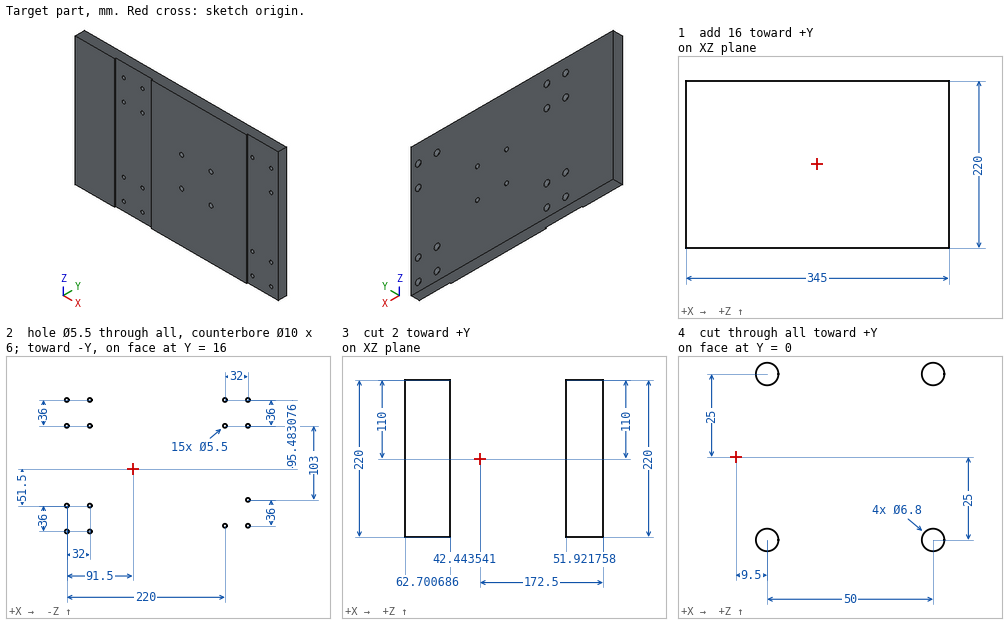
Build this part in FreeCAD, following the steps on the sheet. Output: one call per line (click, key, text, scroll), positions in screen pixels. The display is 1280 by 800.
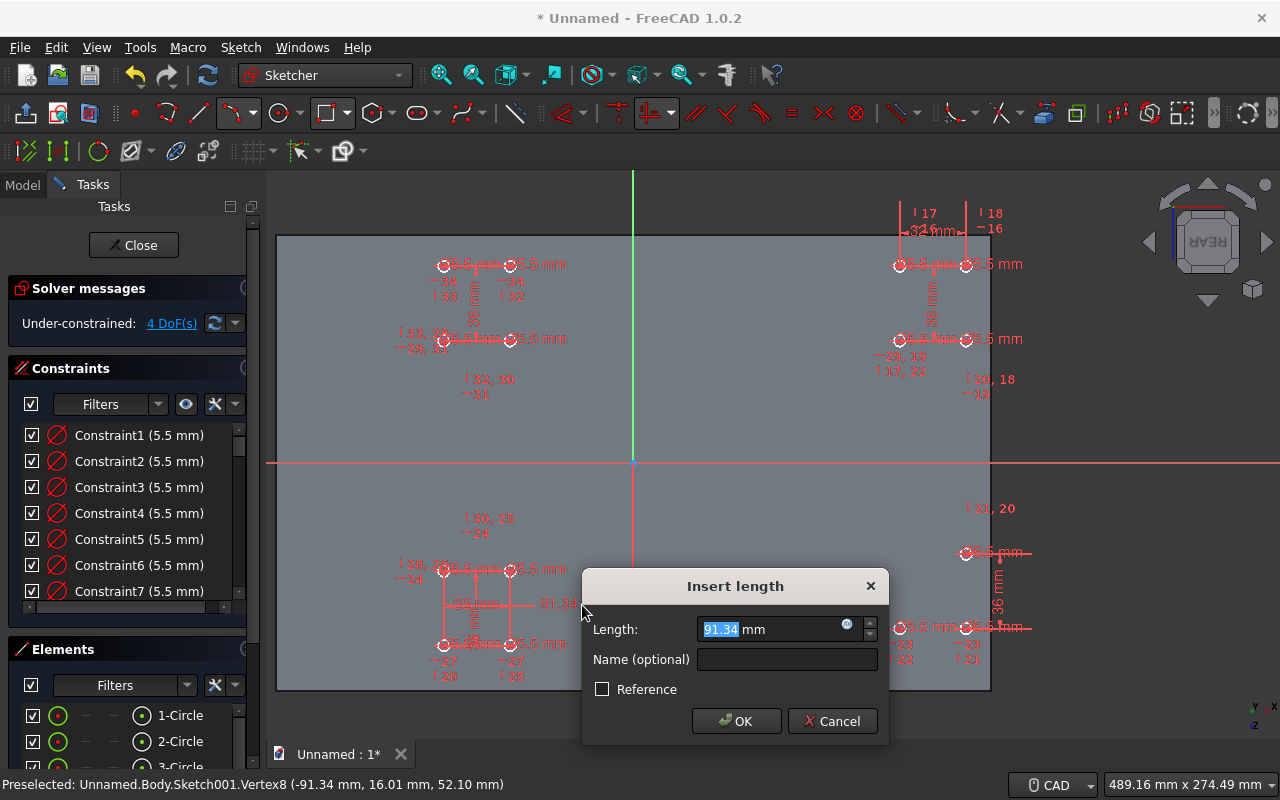
text(91.5)
key(Return)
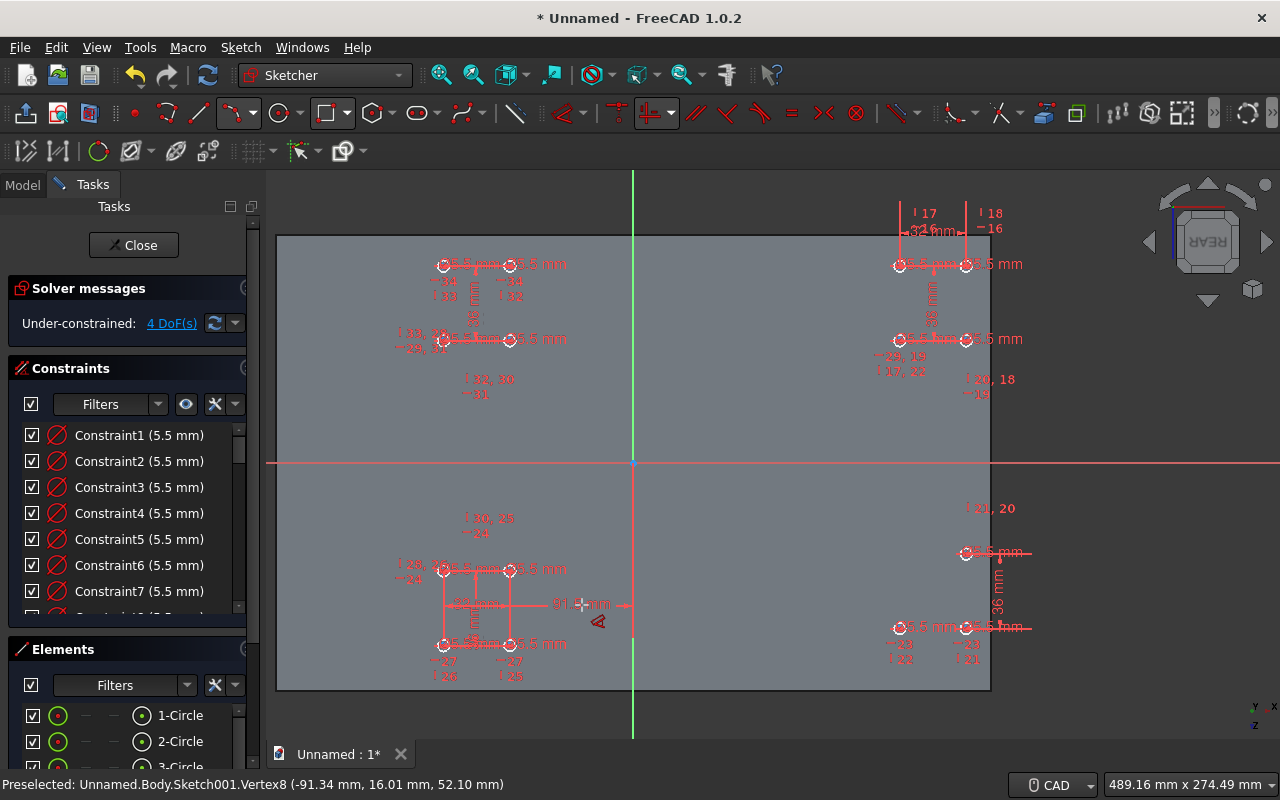
click(444, 571)
click(410, 517)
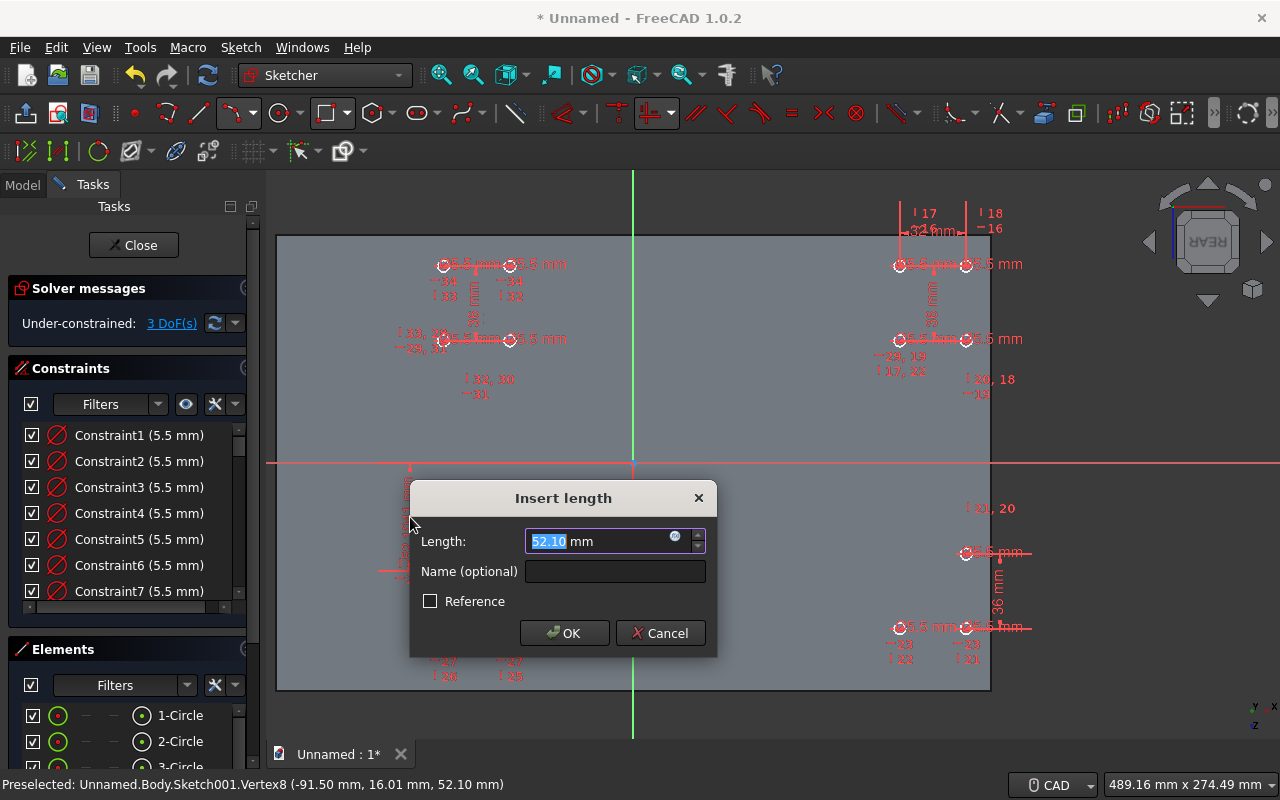
text(51.5)
key(Return)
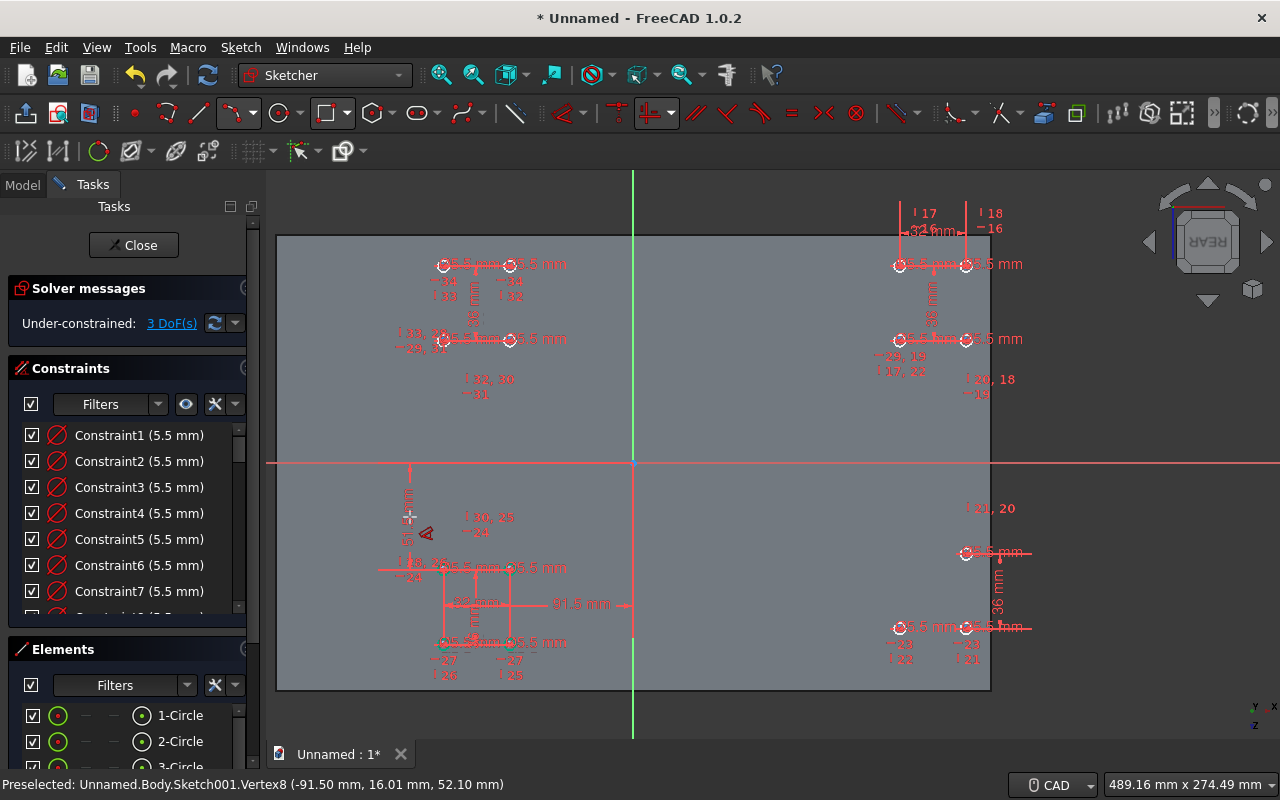
click(966, 341)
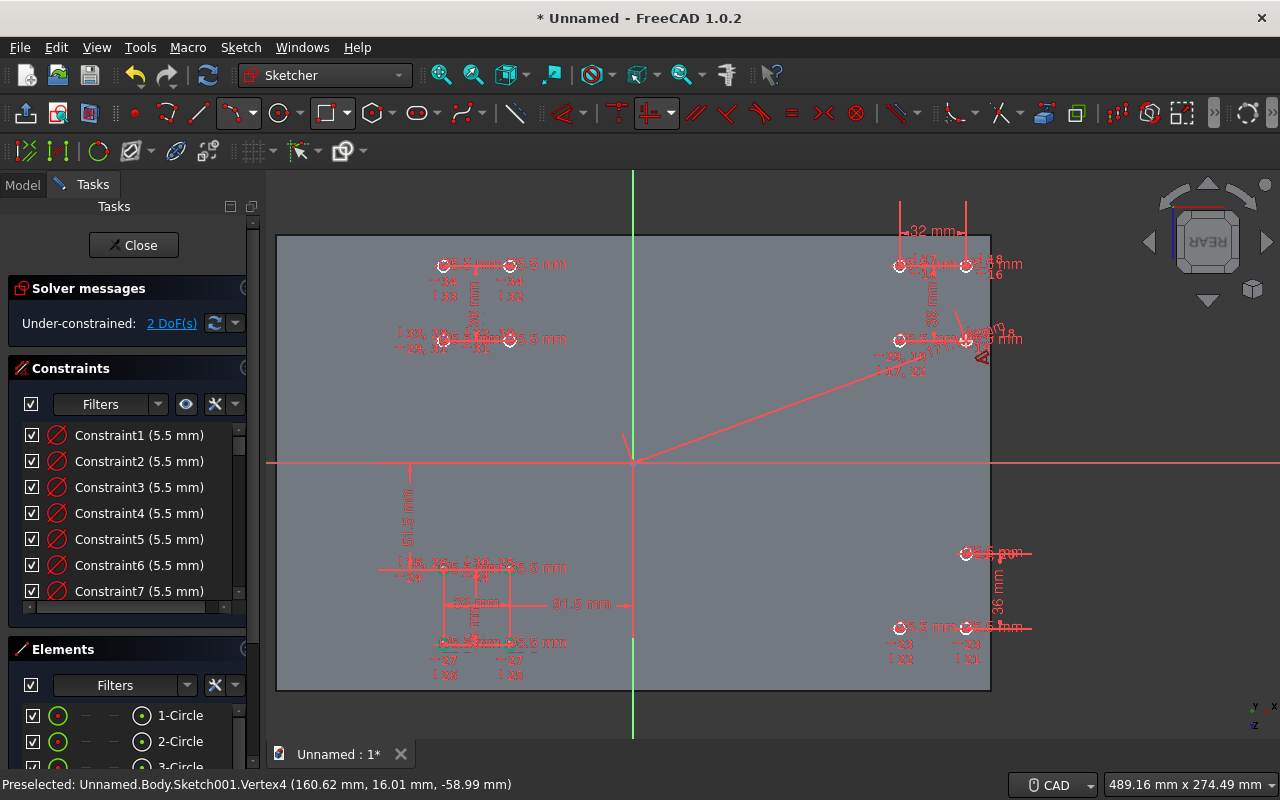
click(966, 554)
click(1000, 447)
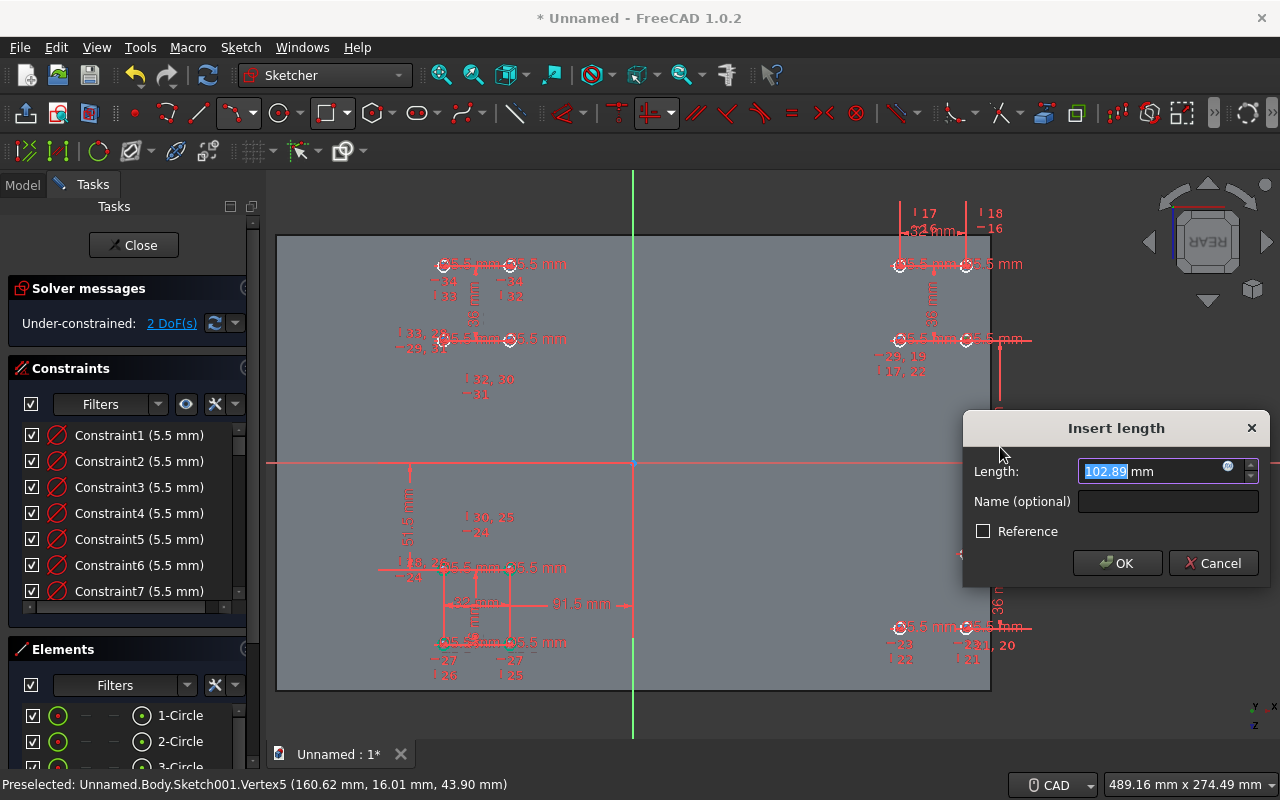
text(103)
key(Return)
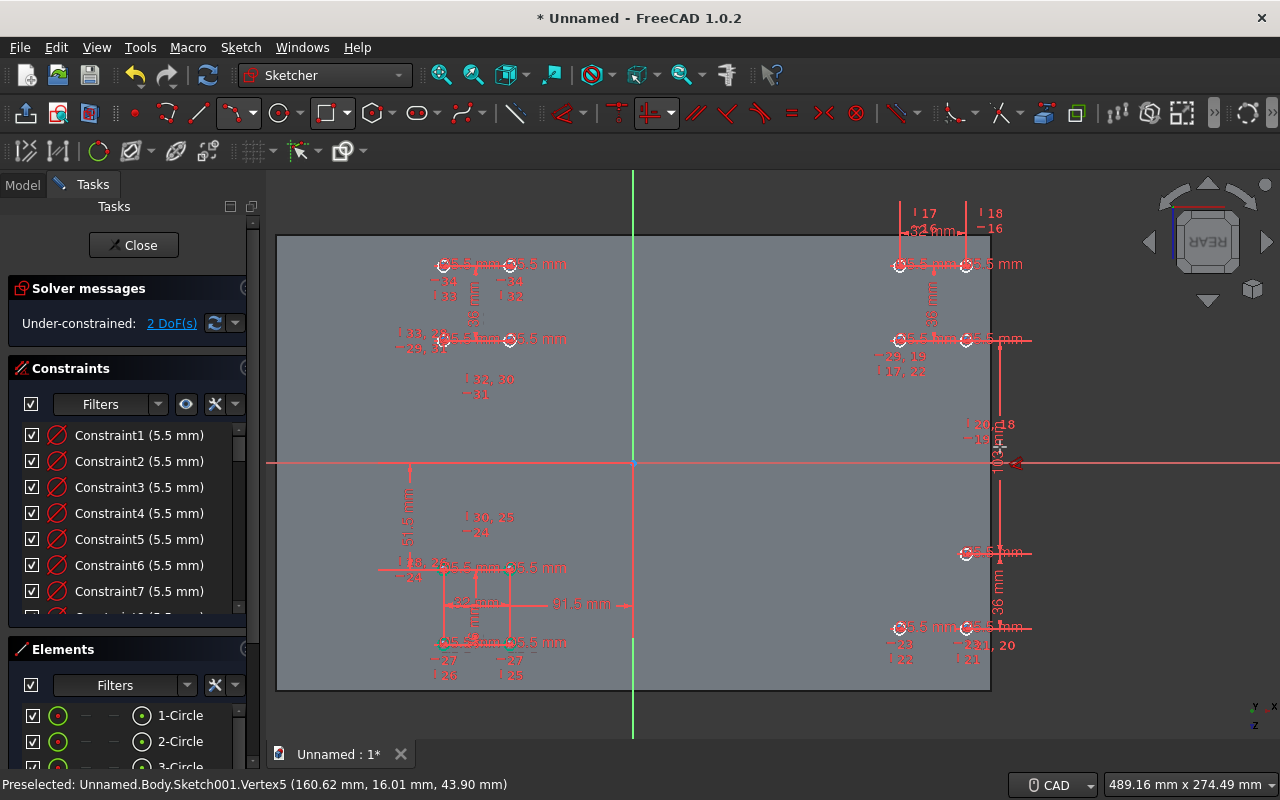
click(900, 629)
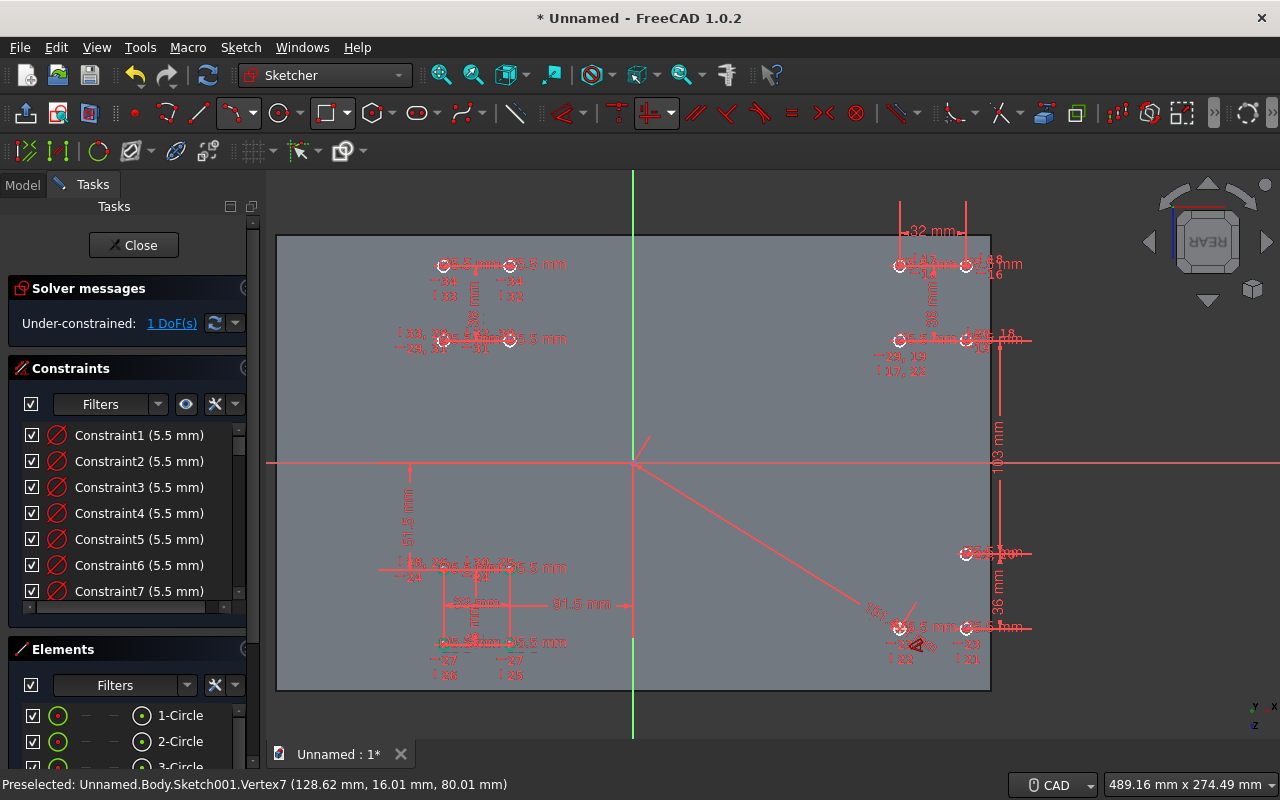
click(444, 570)
click(672, 663)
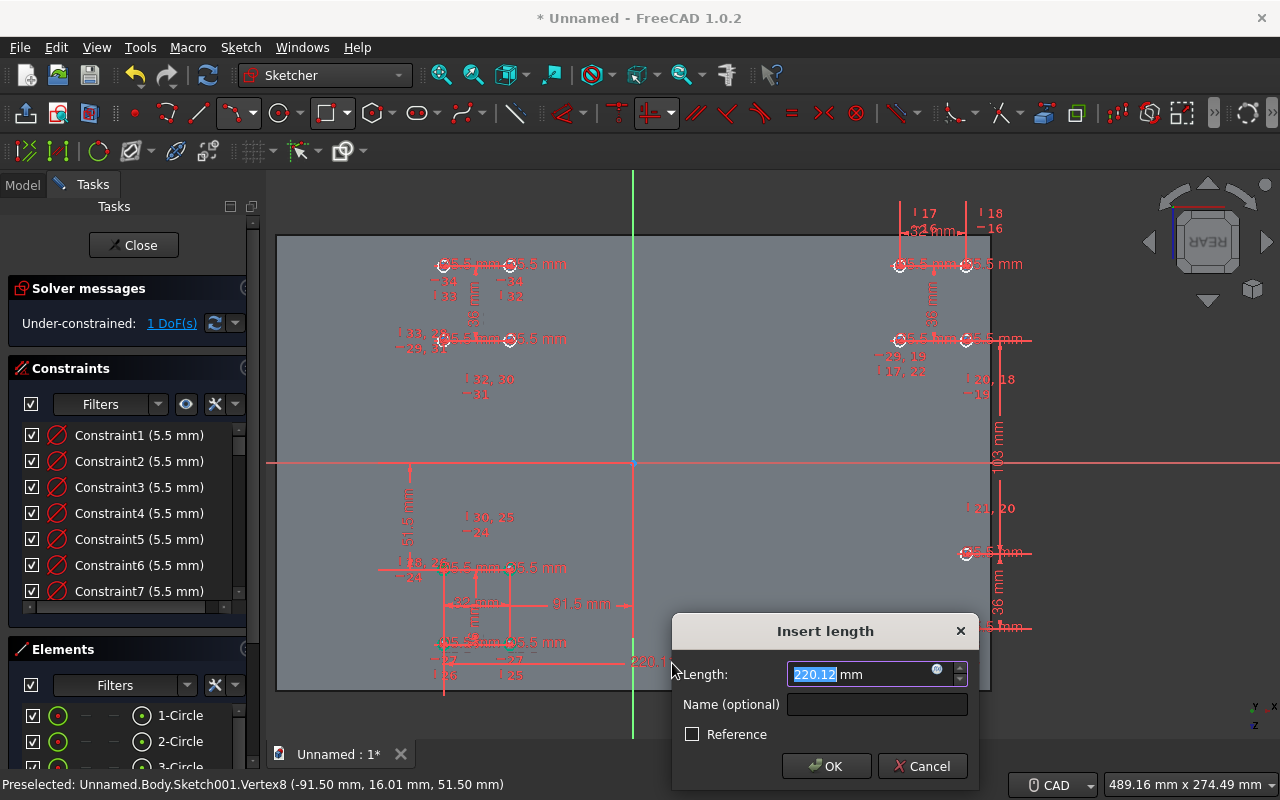
text(220)
key(Return)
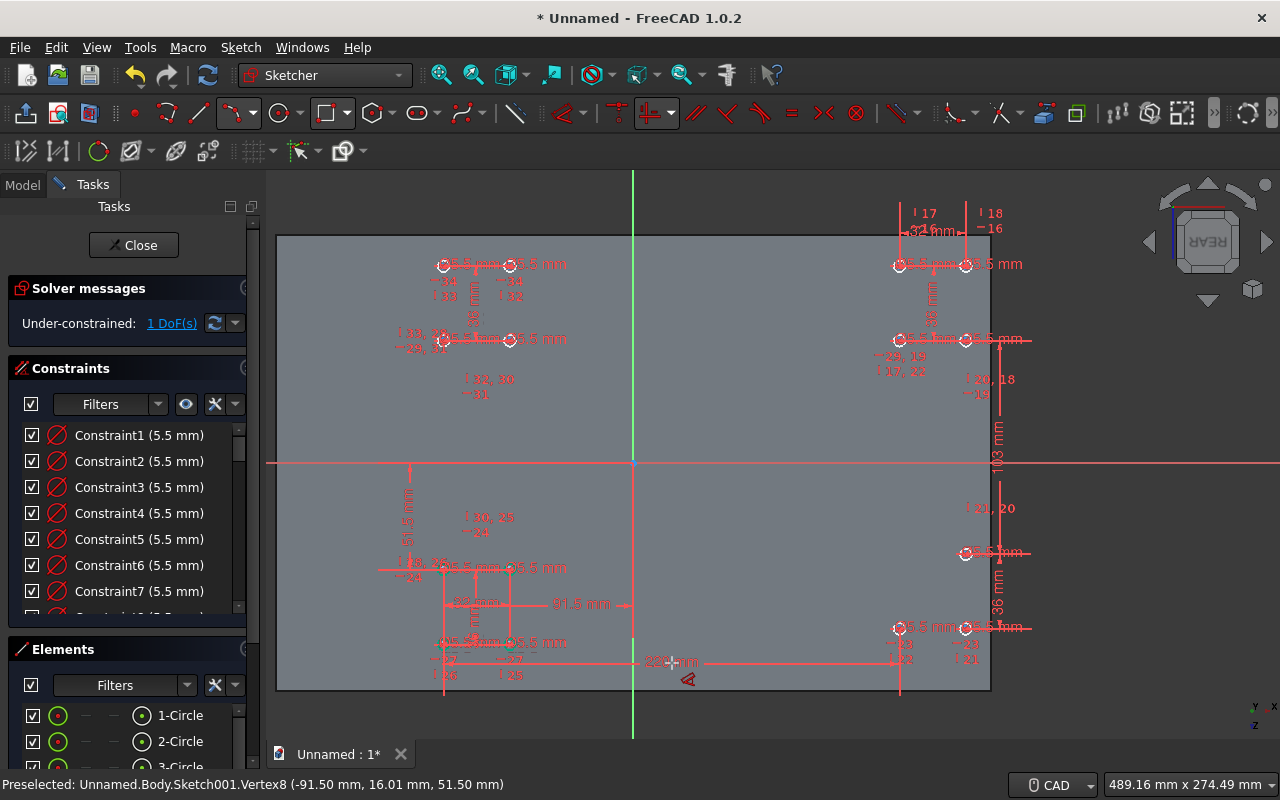
click(966, 266)
click(1000, 365)